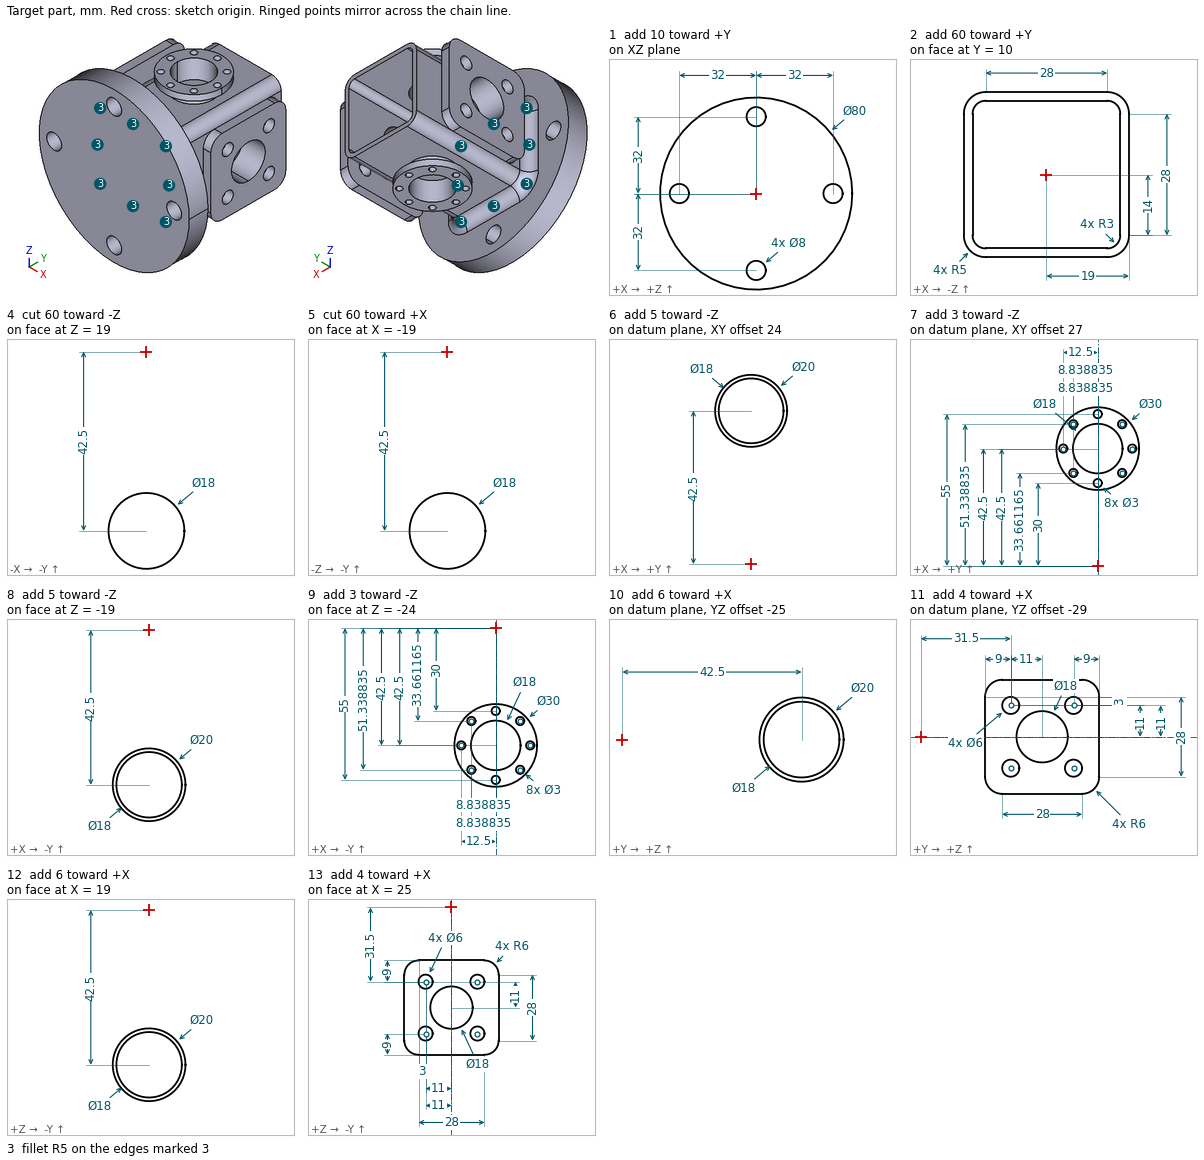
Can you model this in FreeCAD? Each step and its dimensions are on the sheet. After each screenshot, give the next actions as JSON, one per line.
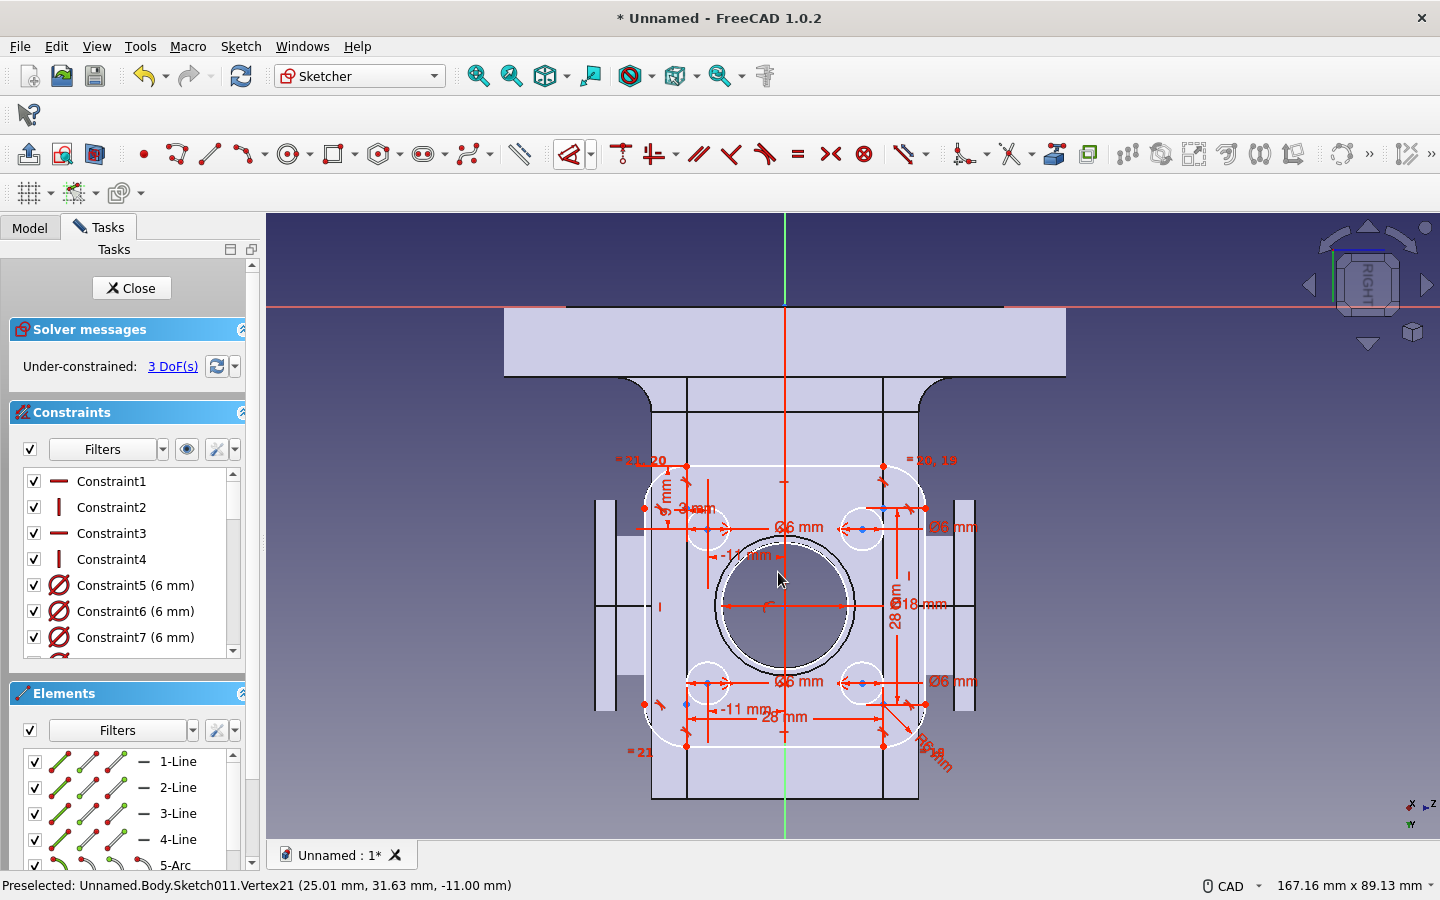
{"action": "left_click", "coordinate": [687, 747]}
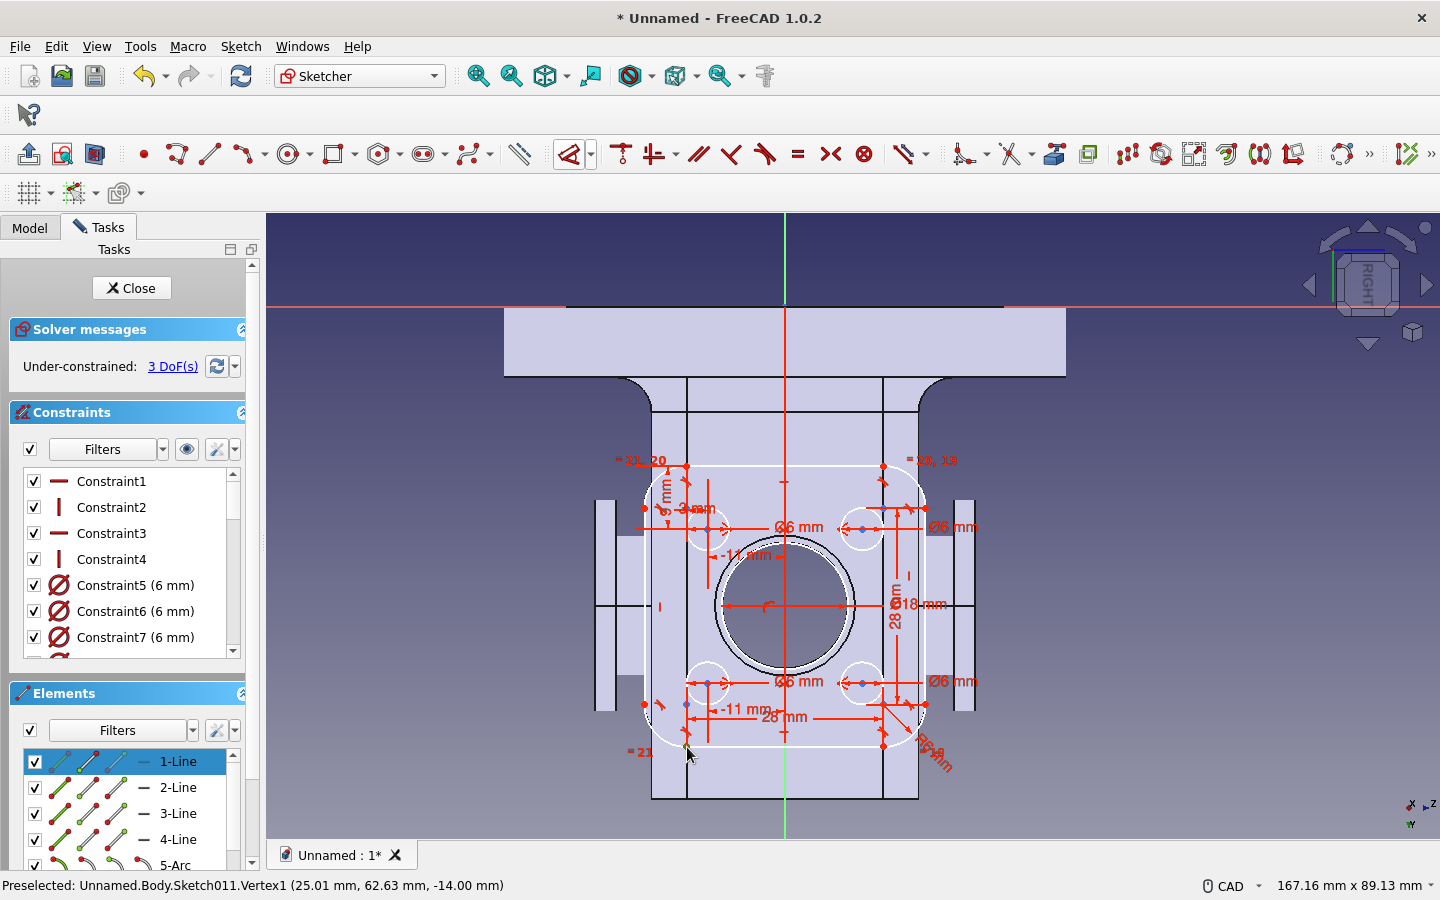
{"action": "left_click", "coordinate": [708, 683]}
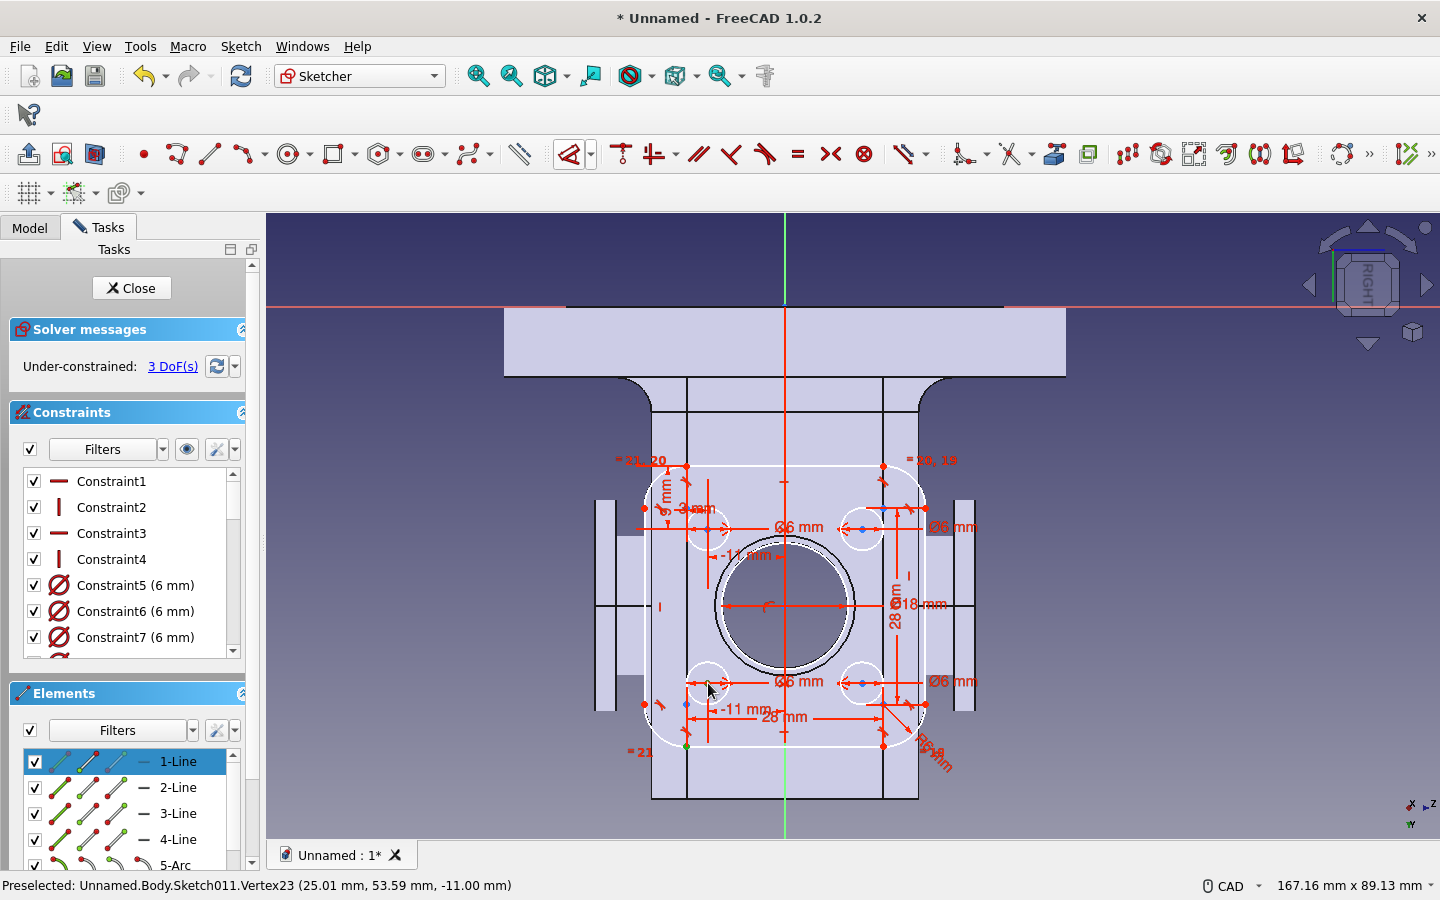
{"action": "key", "text": "i"}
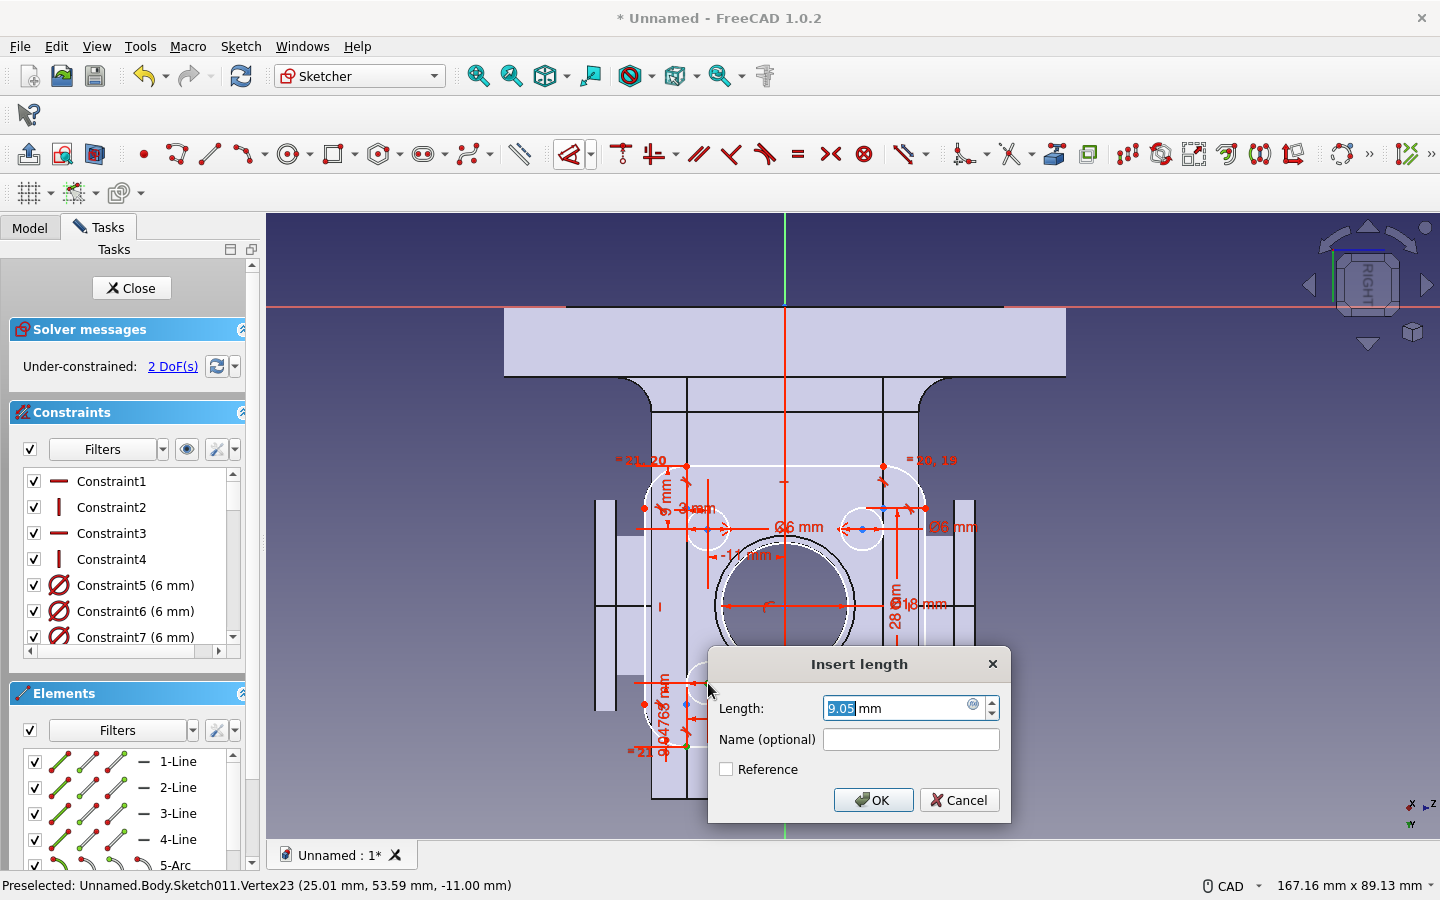
{"action": "type", "text": "9"}
{"action": "key", "text": "Return"}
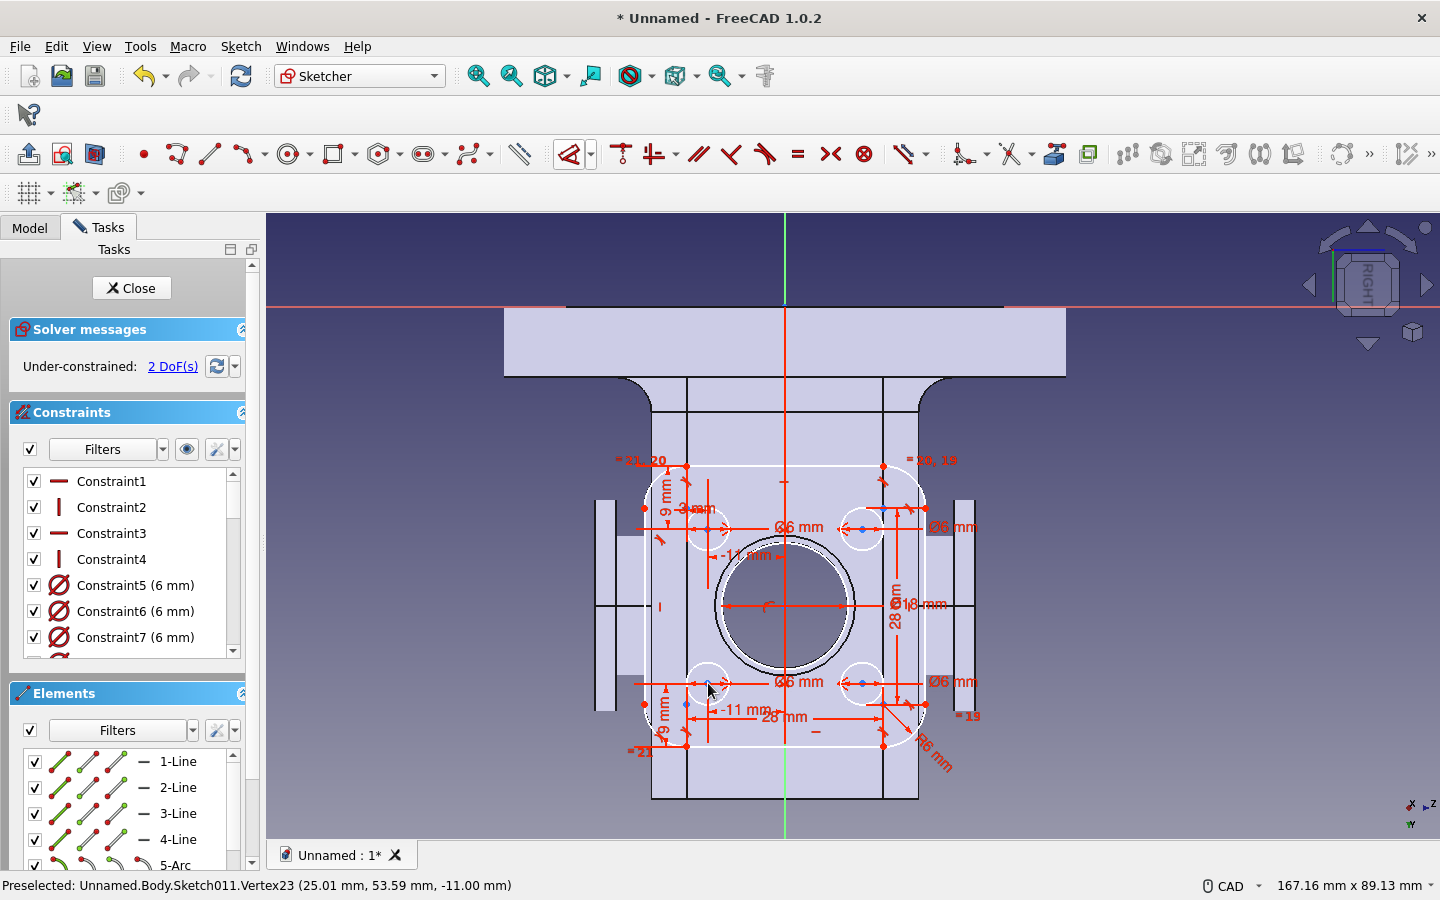
{"action": "left_click", "coordinate": [708, 529]}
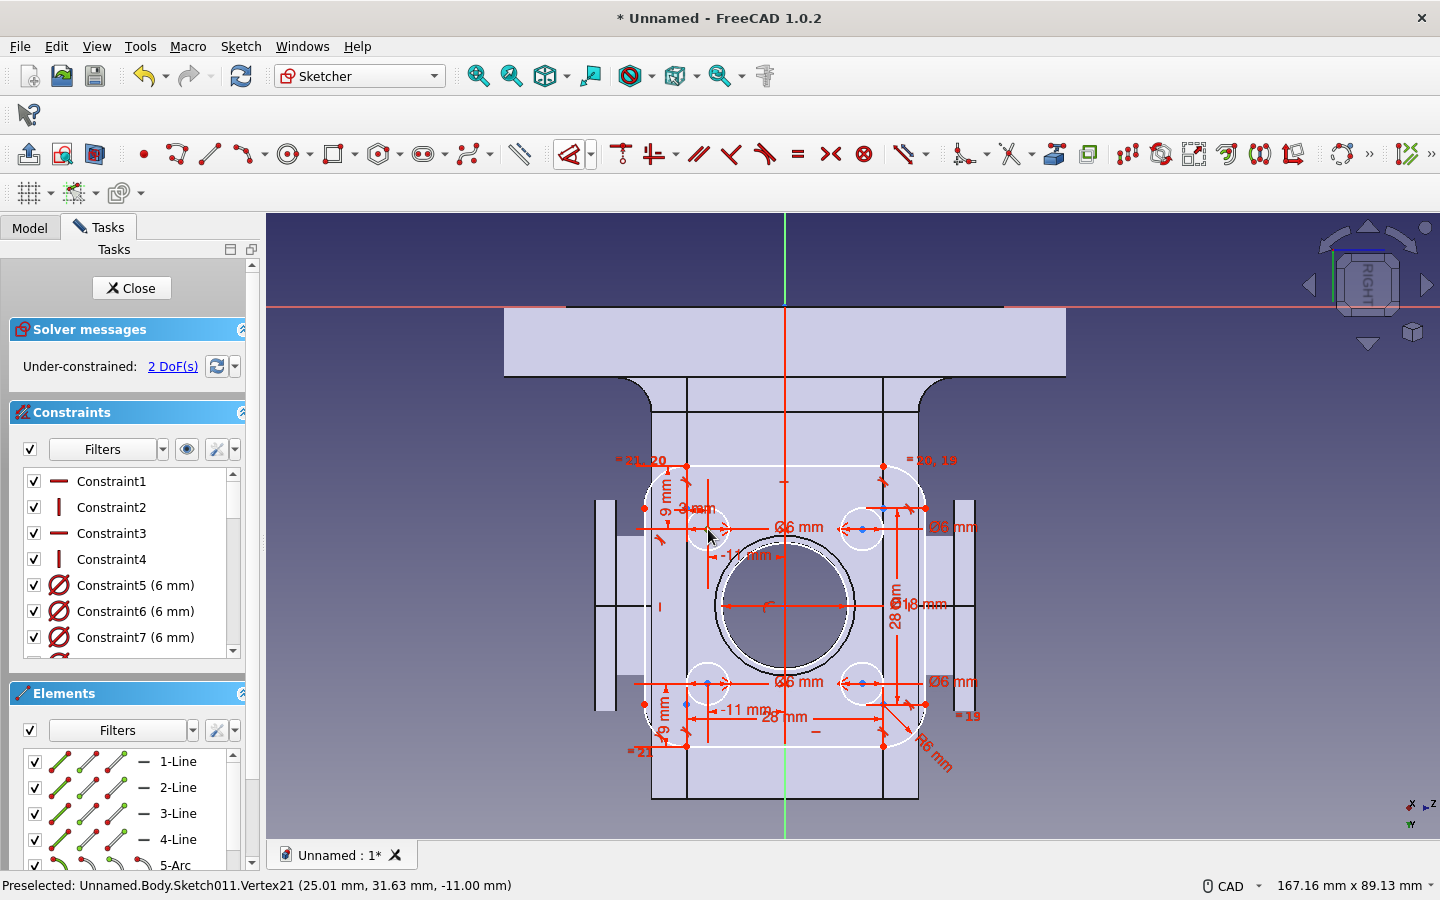
{"action": "left_click", "coordinate": [785, 606]}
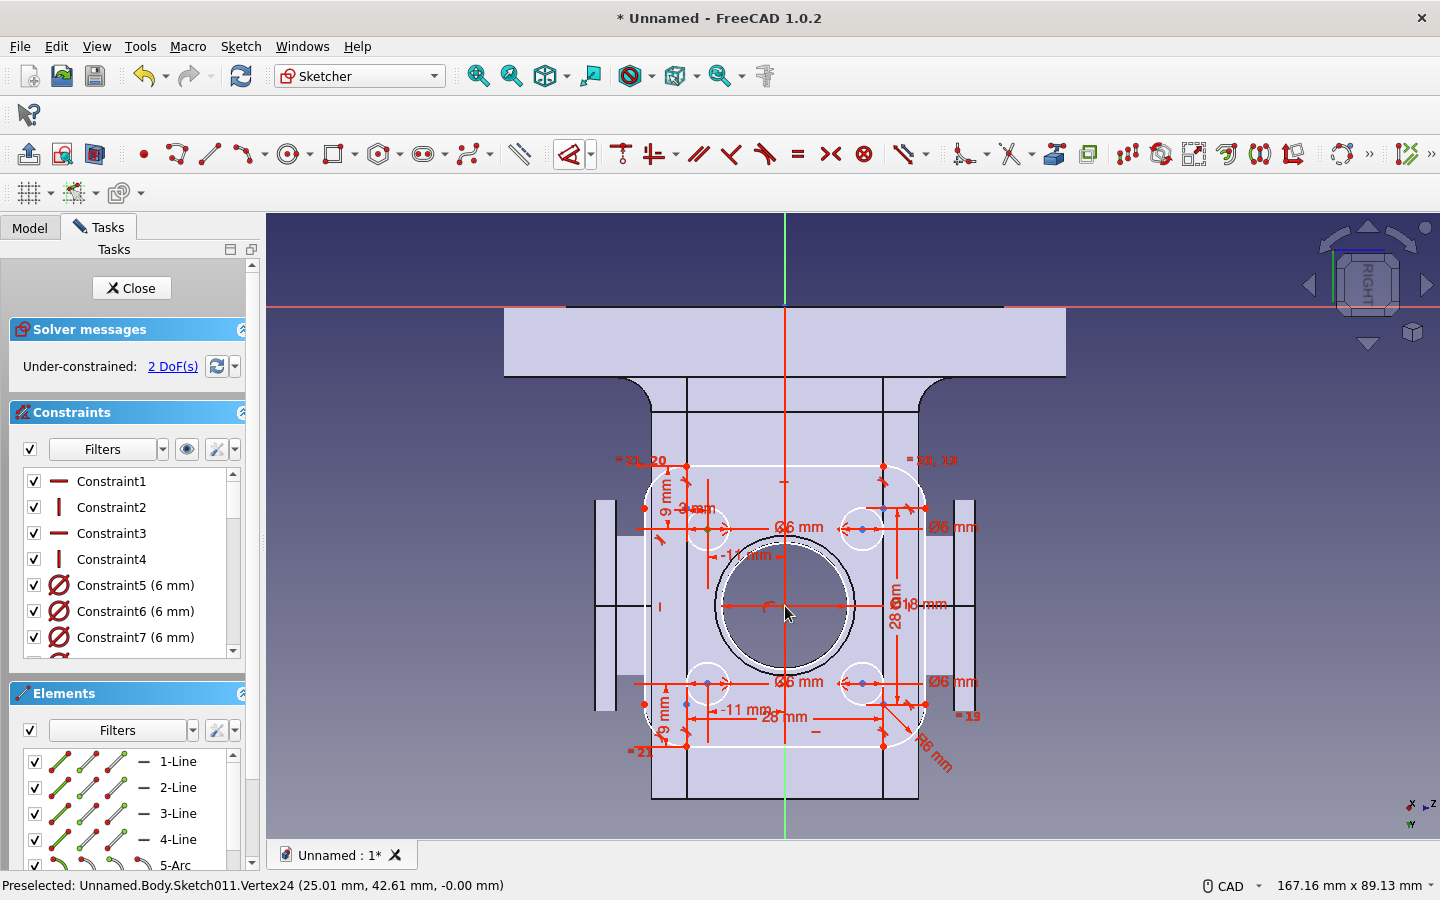
{"action": "key", "text": "i"}